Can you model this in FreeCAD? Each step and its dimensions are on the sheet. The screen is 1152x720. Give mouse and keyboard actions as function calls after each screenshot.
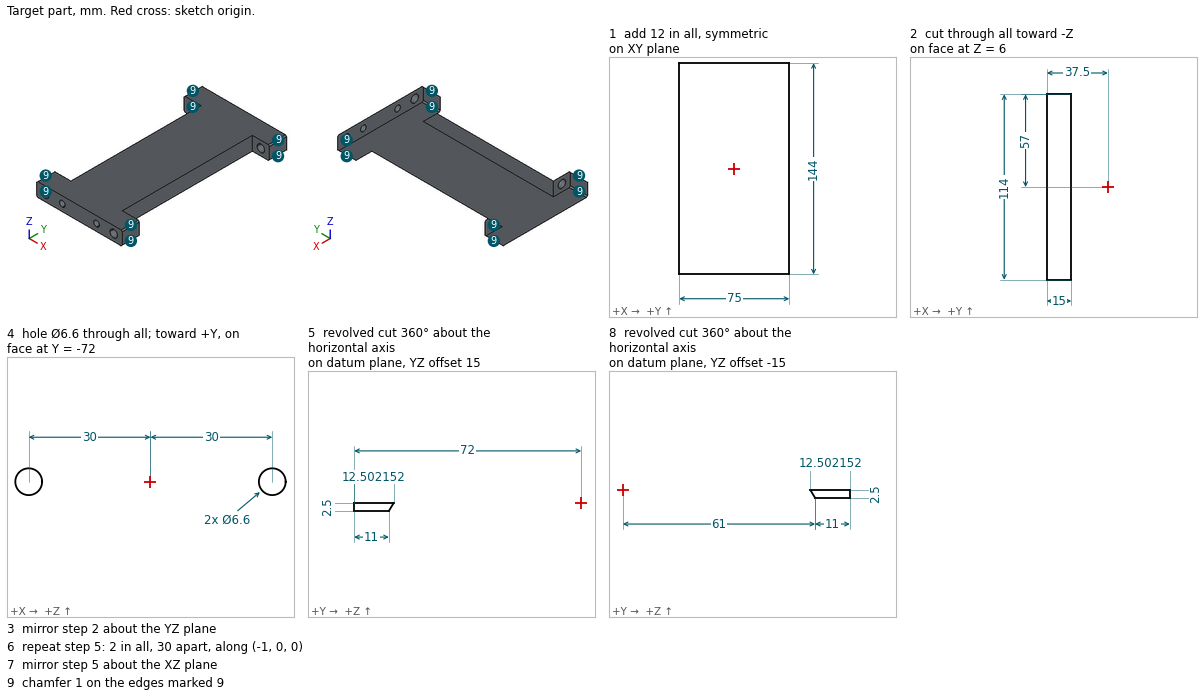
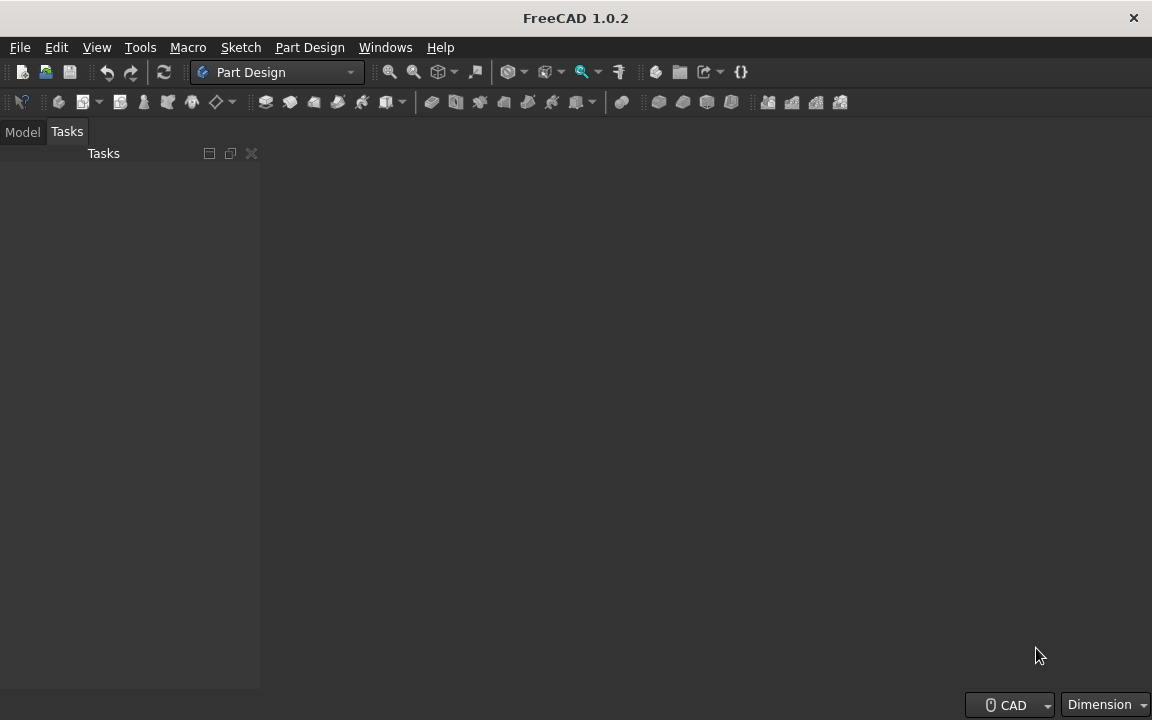
key(ctrl+n)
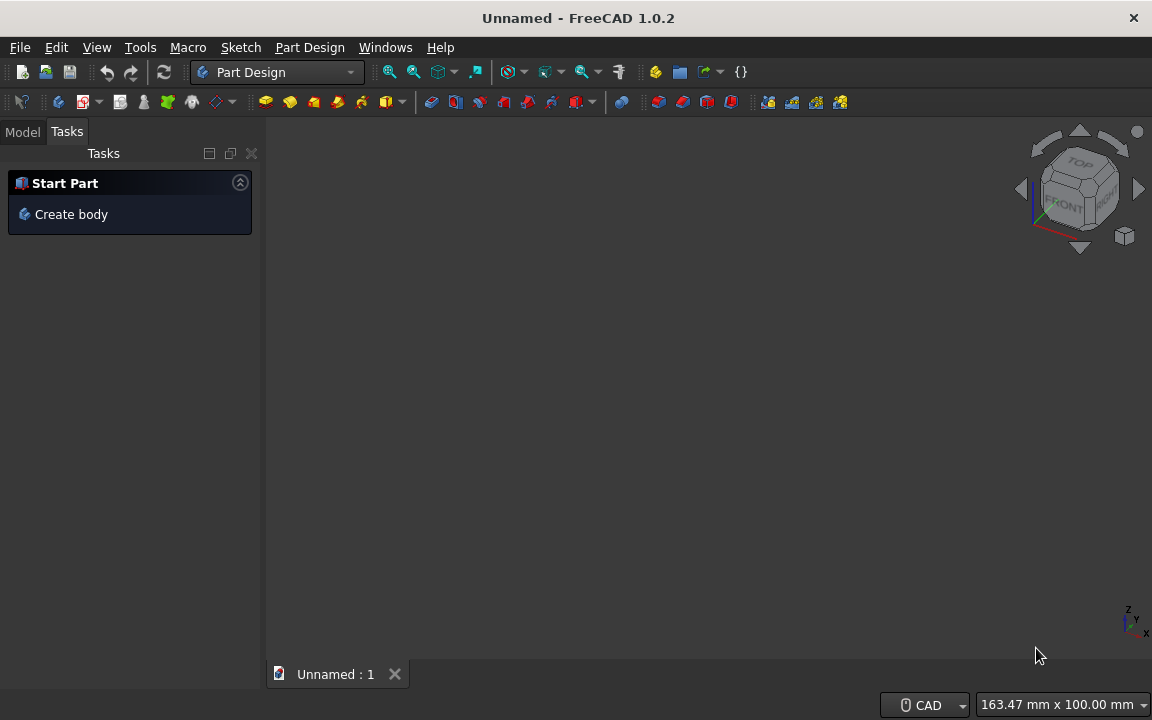
click(84, 102)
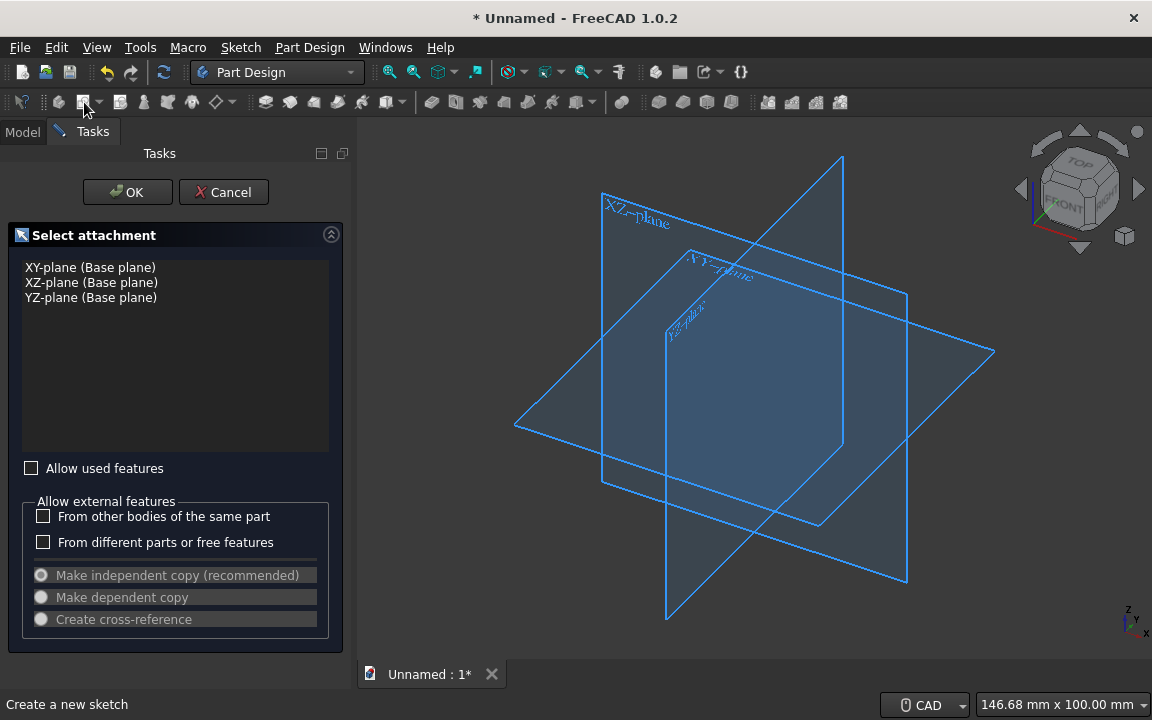
click(82, 268)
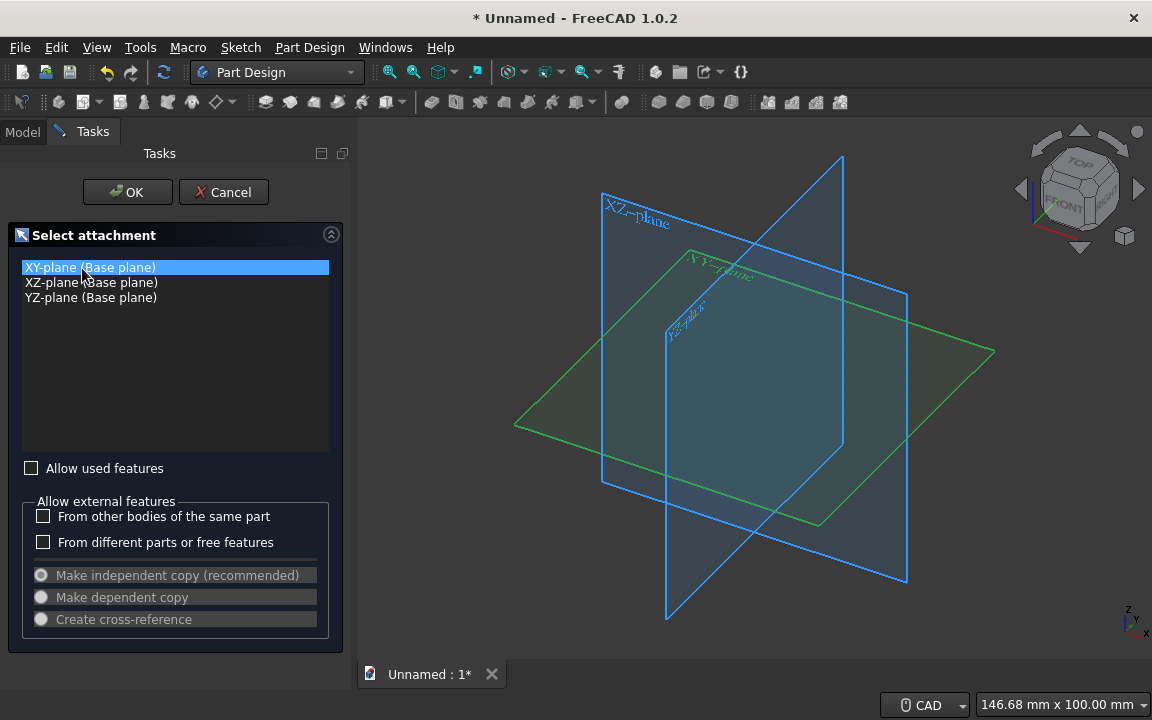
click(128, 192)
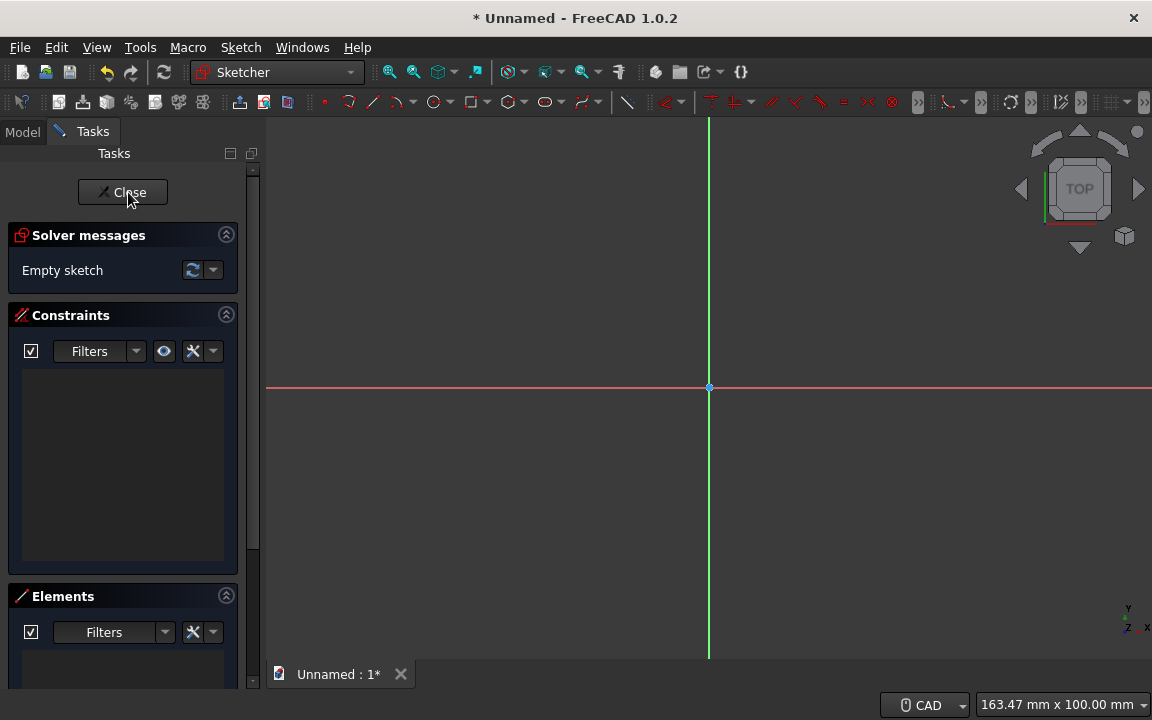
scroll(585, 388, down, 4)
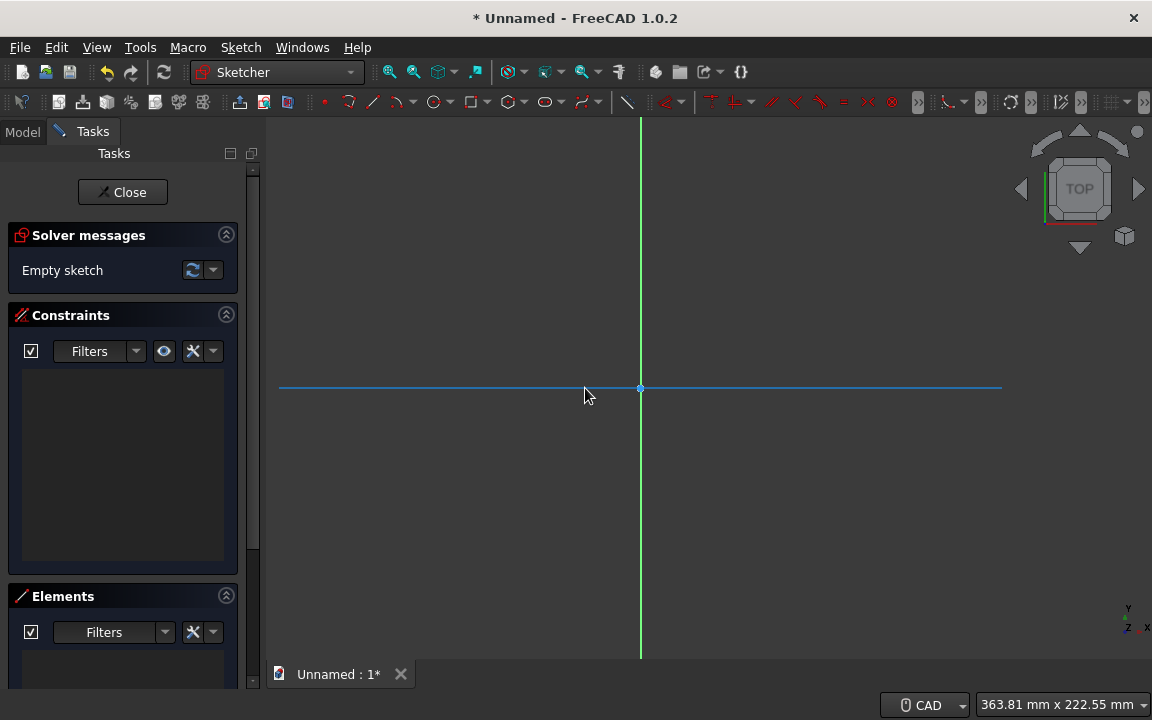
key(g)
key(v)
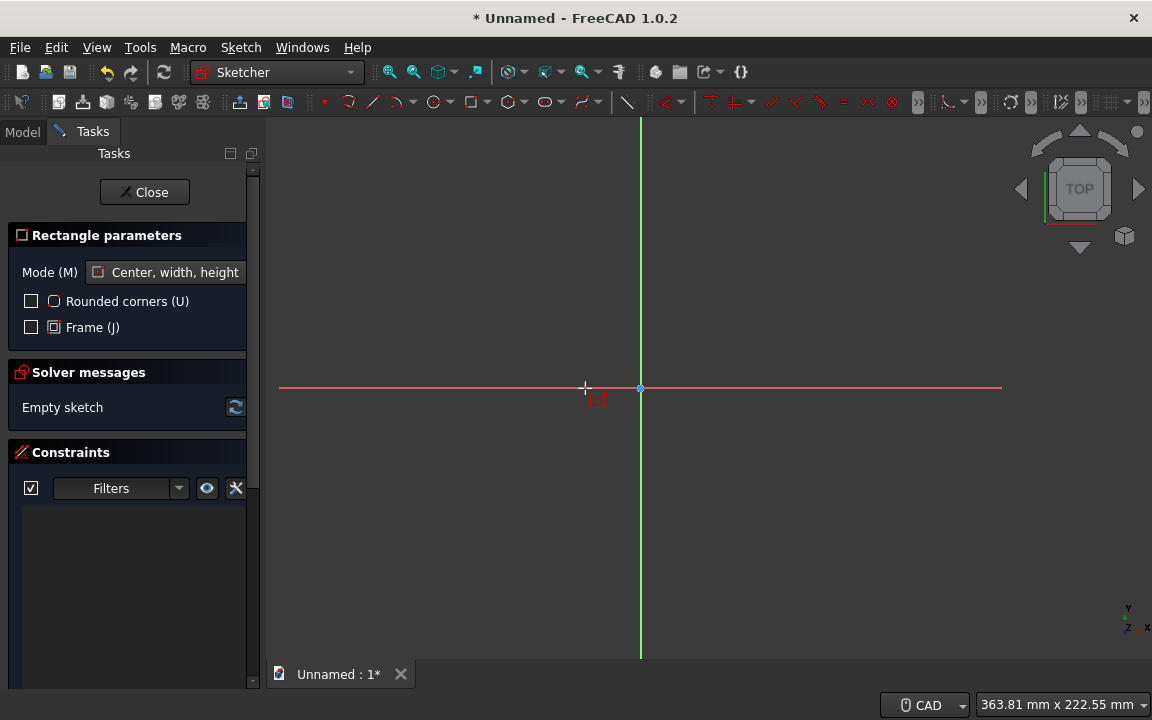
click(641, 388)
move(732, 213)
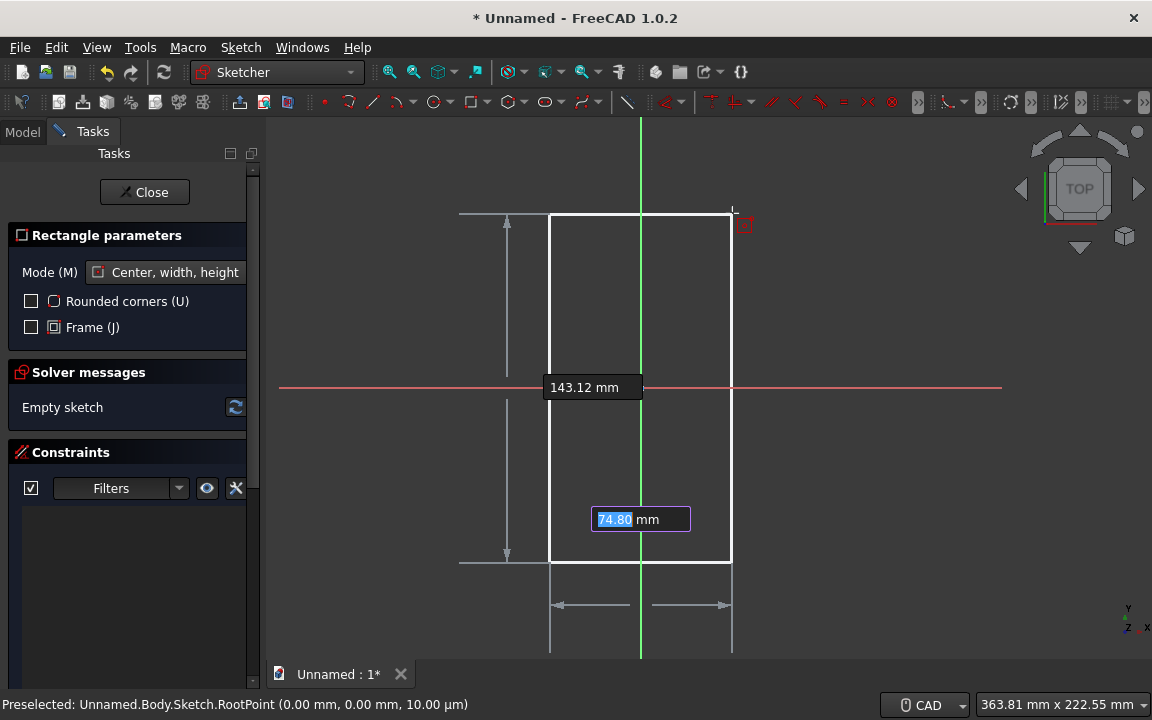
text(75)
key(Tab)
text(144)
key(Return)
key(Escape)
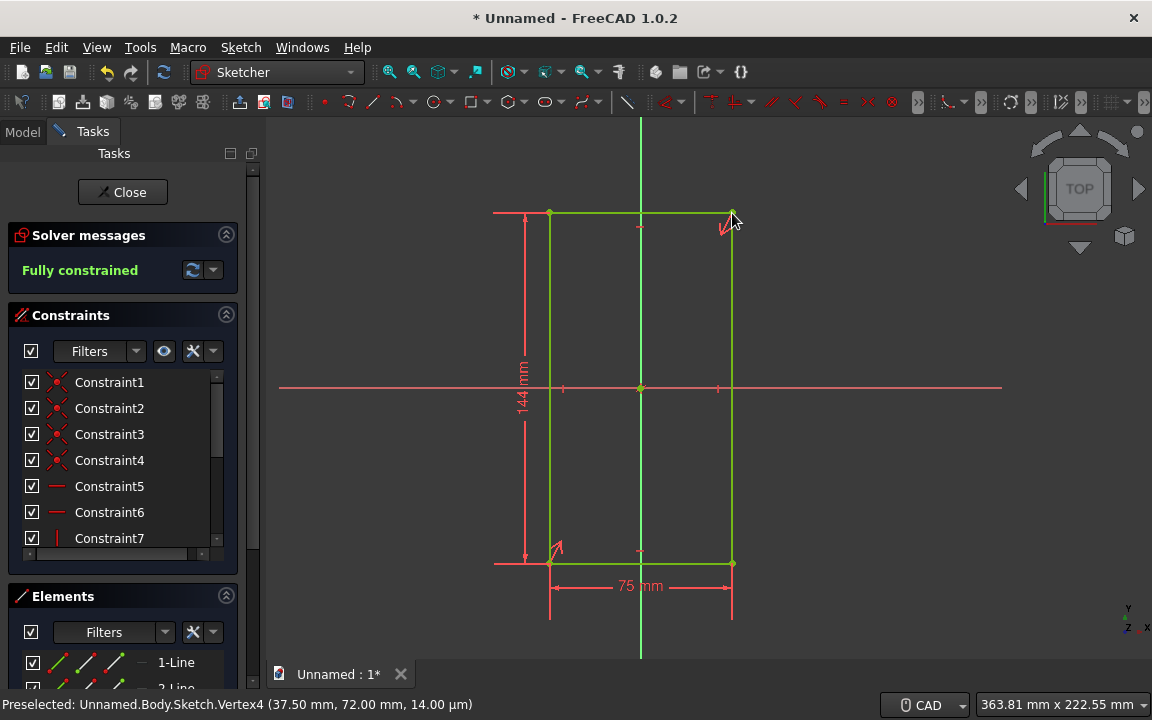
click(123, 192)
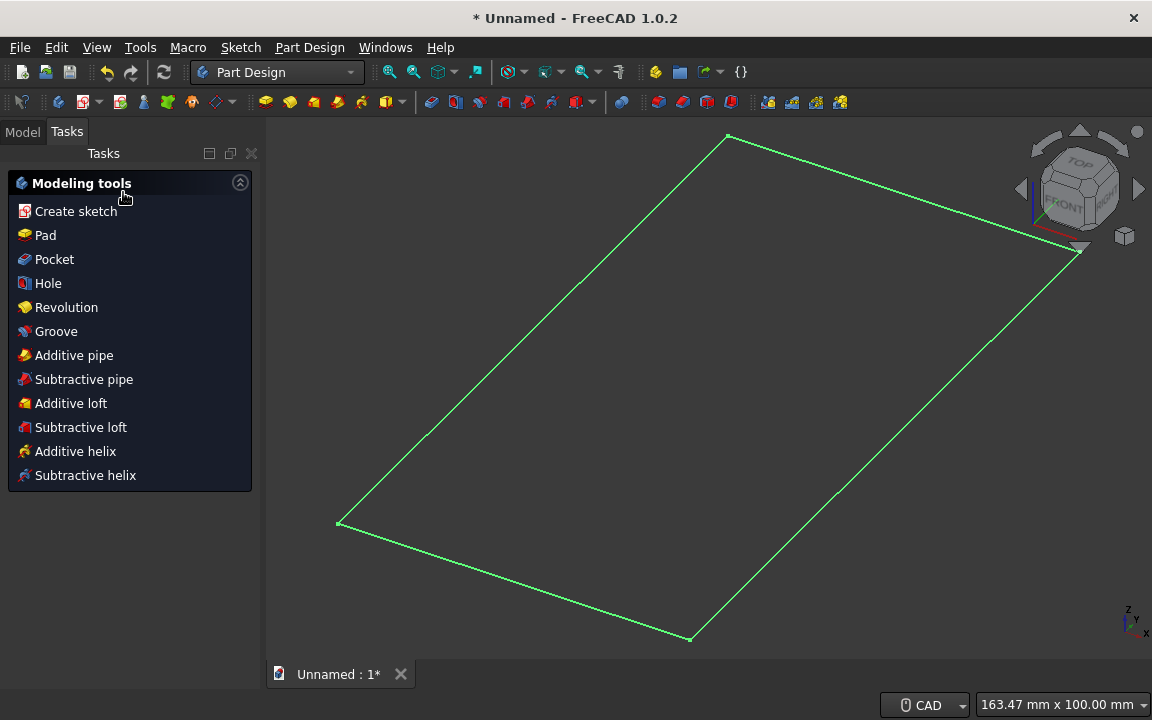
click(266, 102)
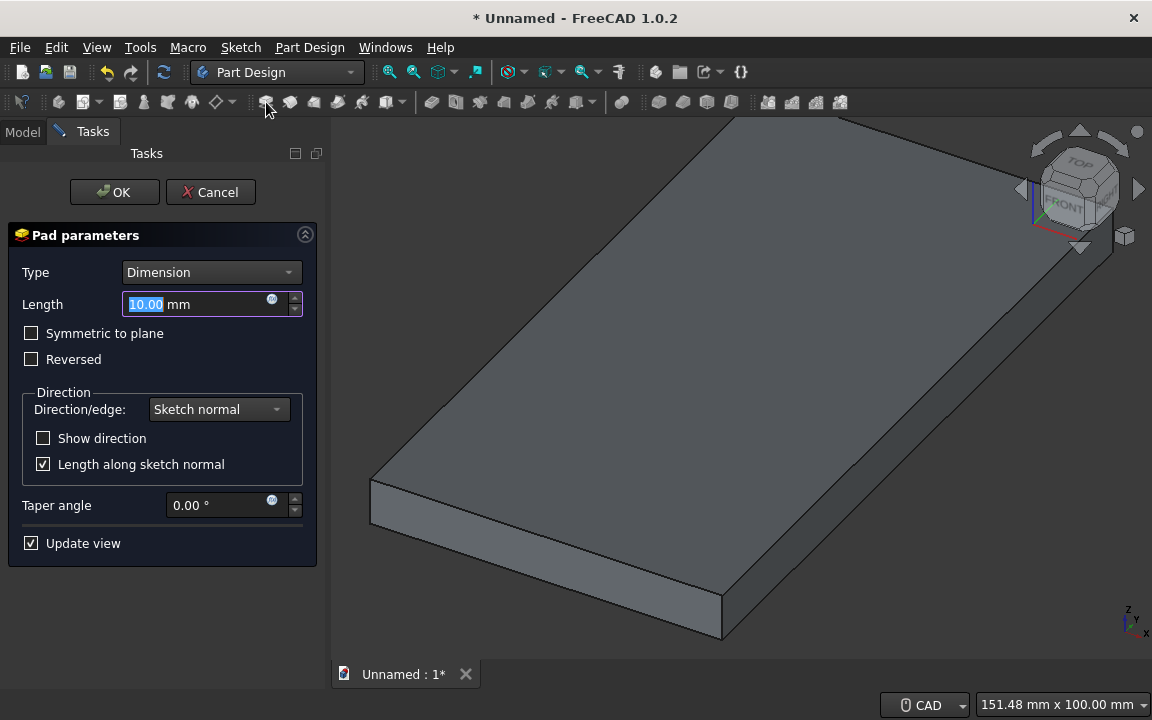
text(12)
key(Tab)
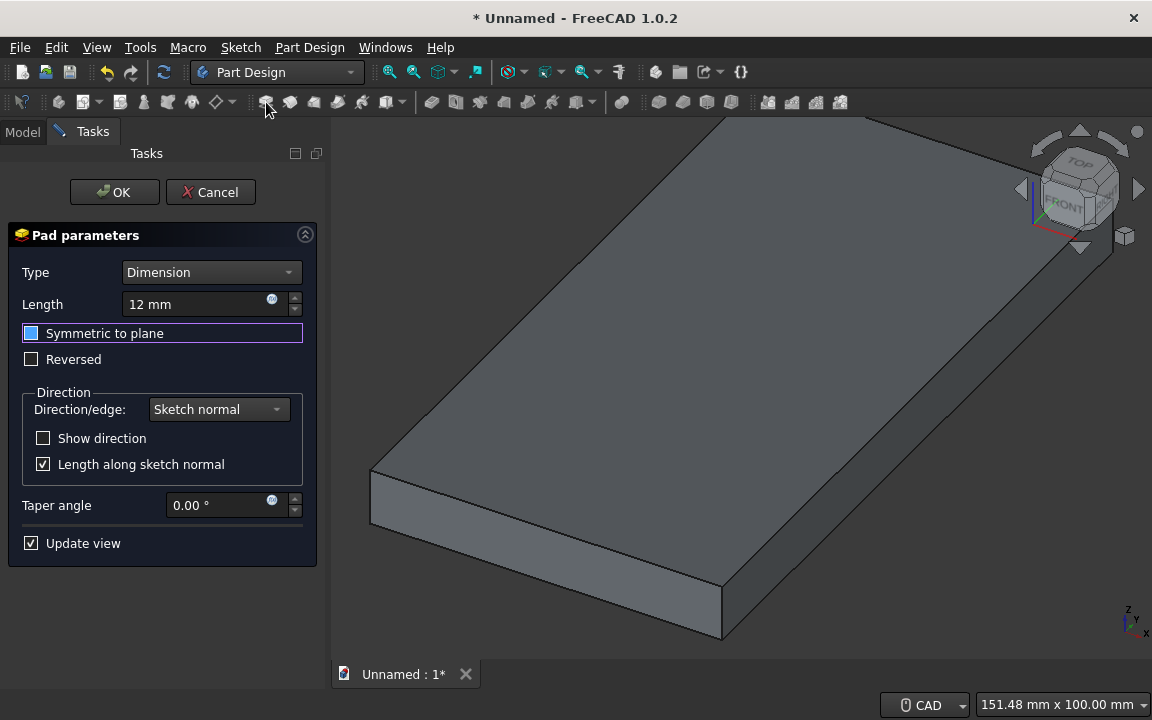
click(30, 333)